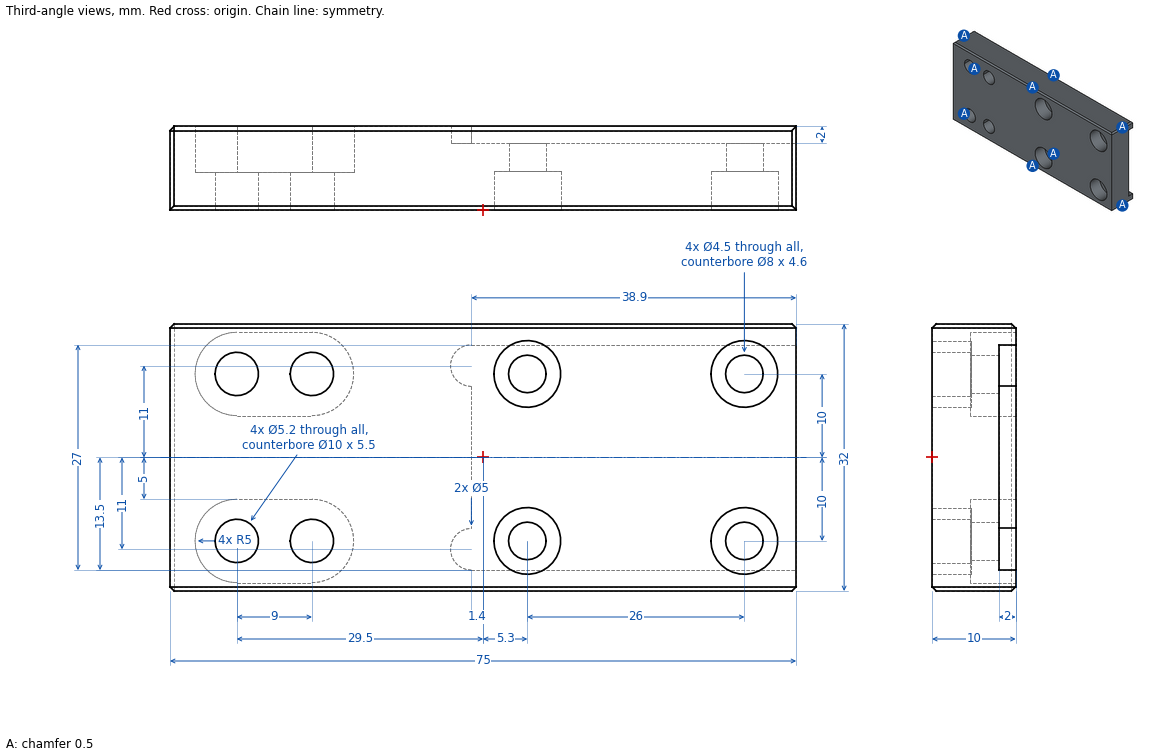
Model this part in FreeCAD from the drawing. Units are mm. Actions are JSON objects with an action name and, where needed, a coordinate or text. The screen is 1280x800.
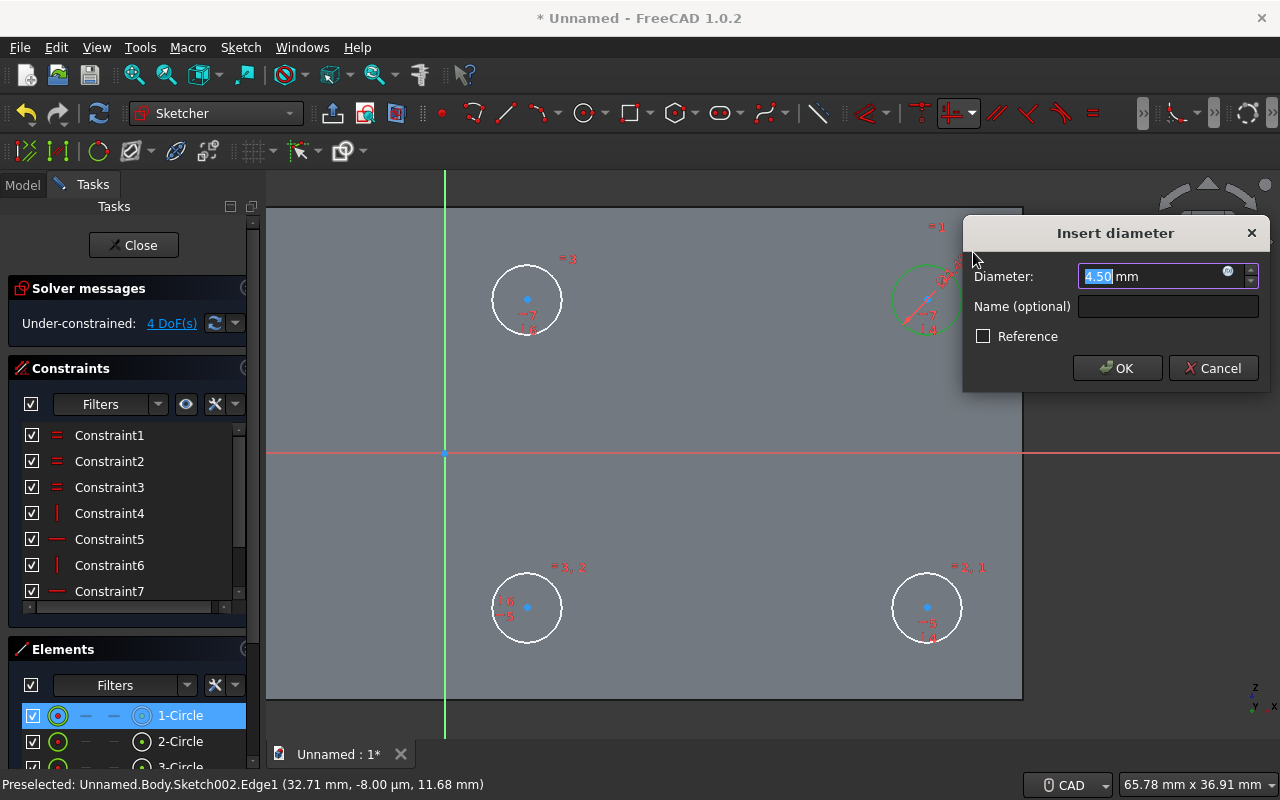
{"action": "type", "text": "4.5"}
{"action": "key", "text": "Return"}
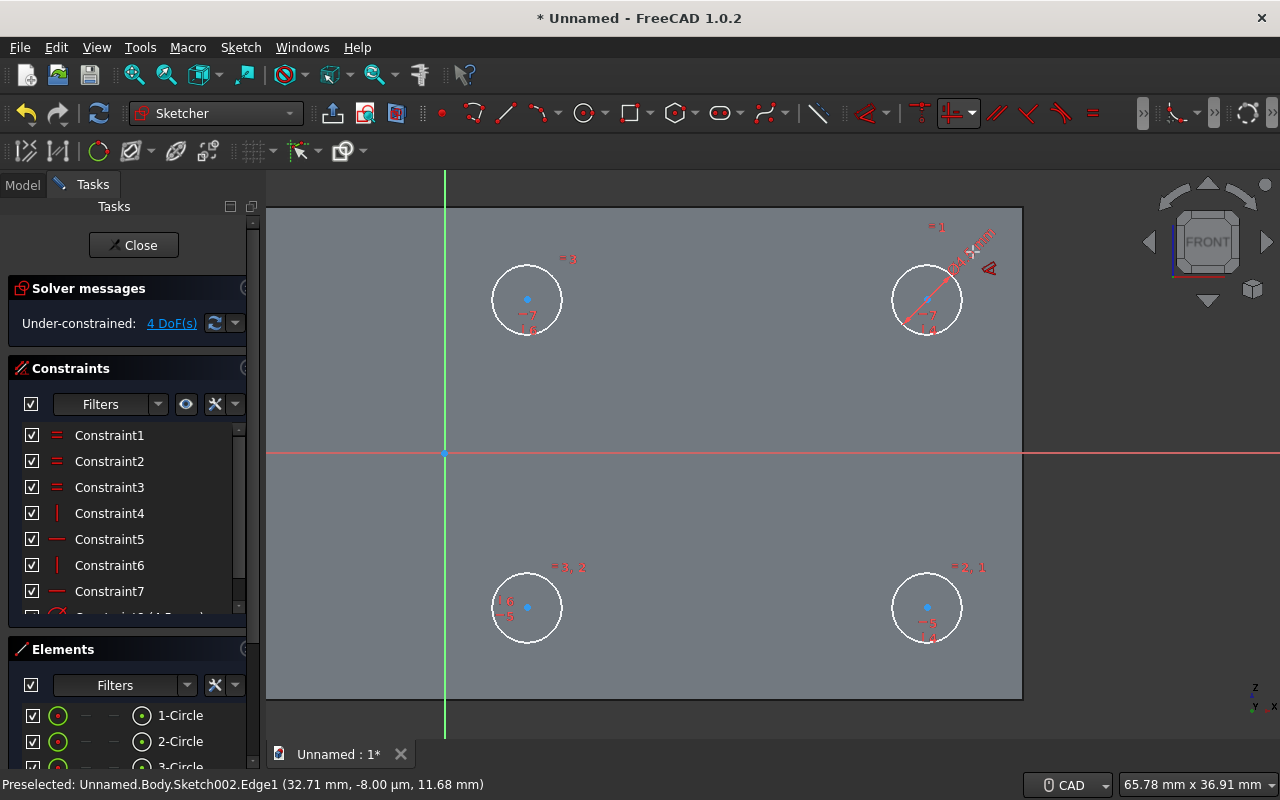
{"action": "left_click", "coordinate": [927, 300]}
{"action": "left_click", "coordinate": [411, 377]}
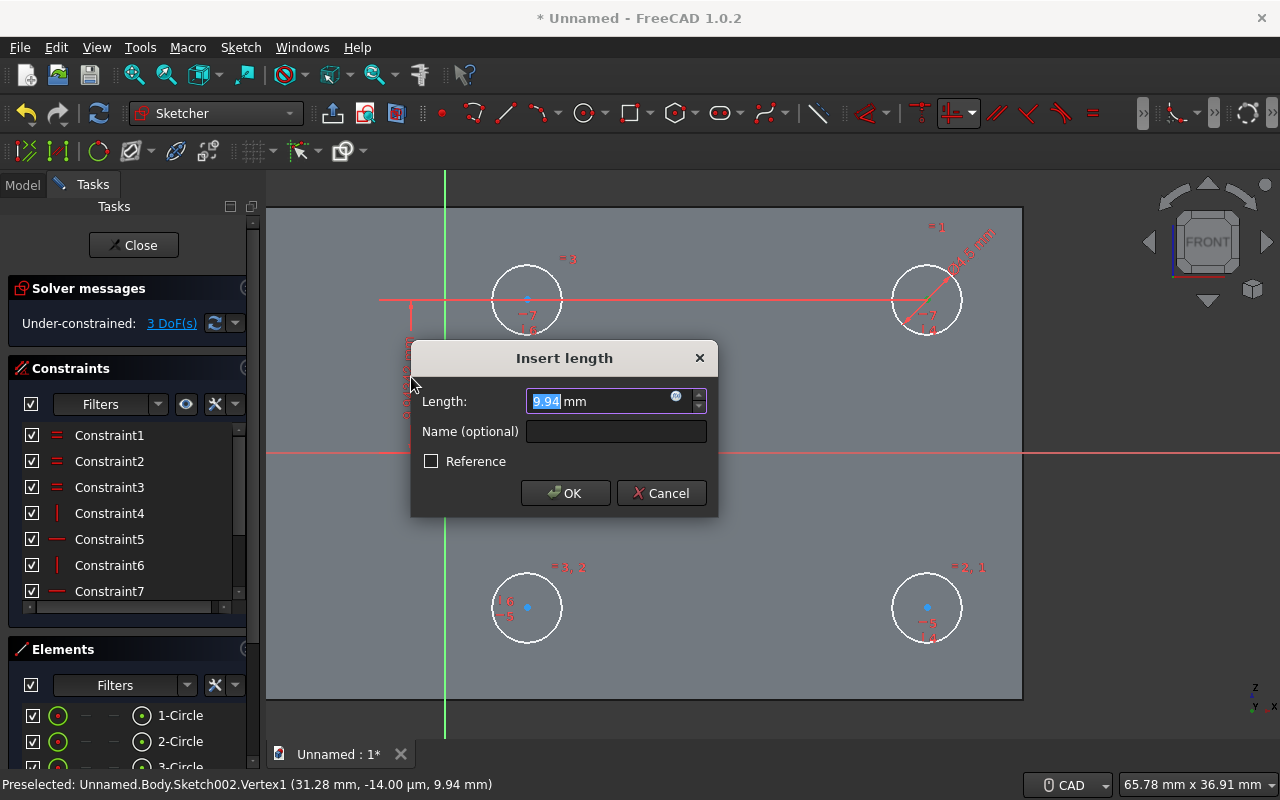
{"action": "type", "text": "10"}
{"action": "key", "text": "Return"}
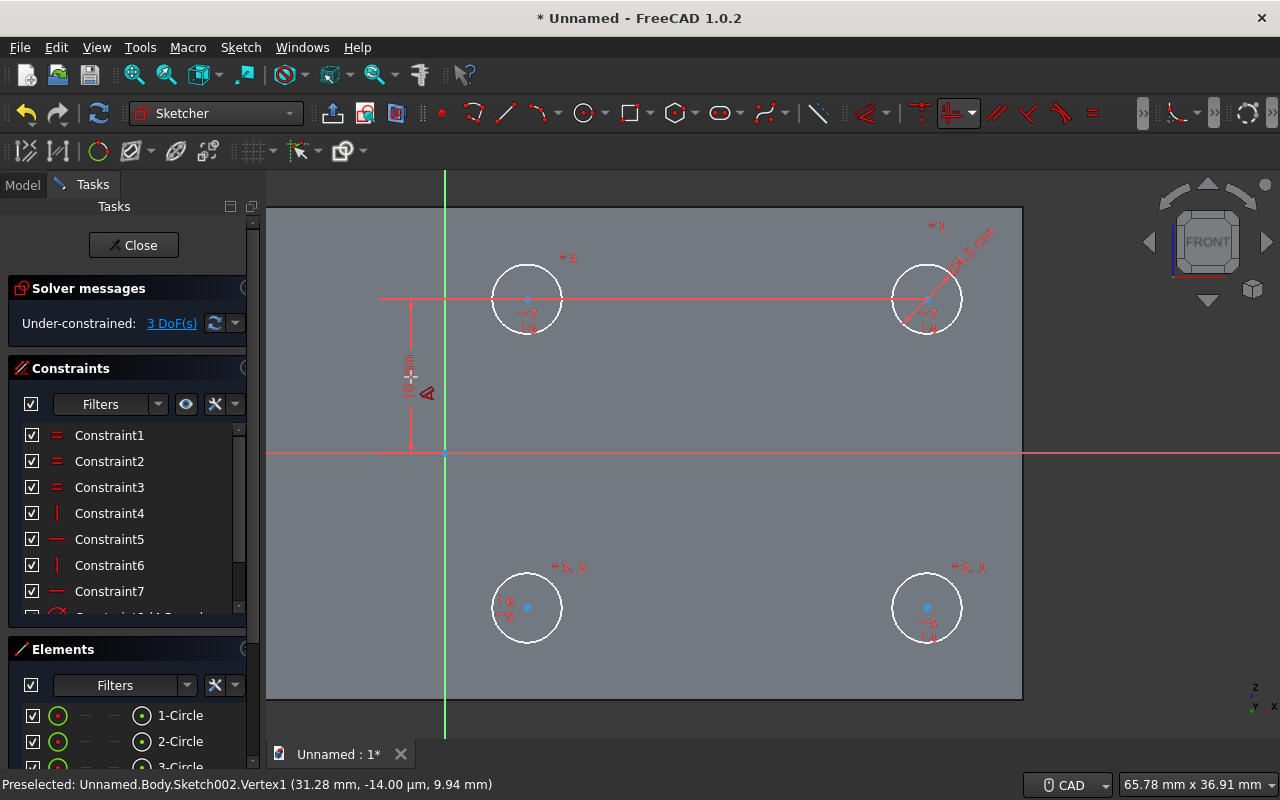
{"action": "left_click", "coordinate": [927, 608]}
{"action": "left_click", "coordinate": [411, 531]}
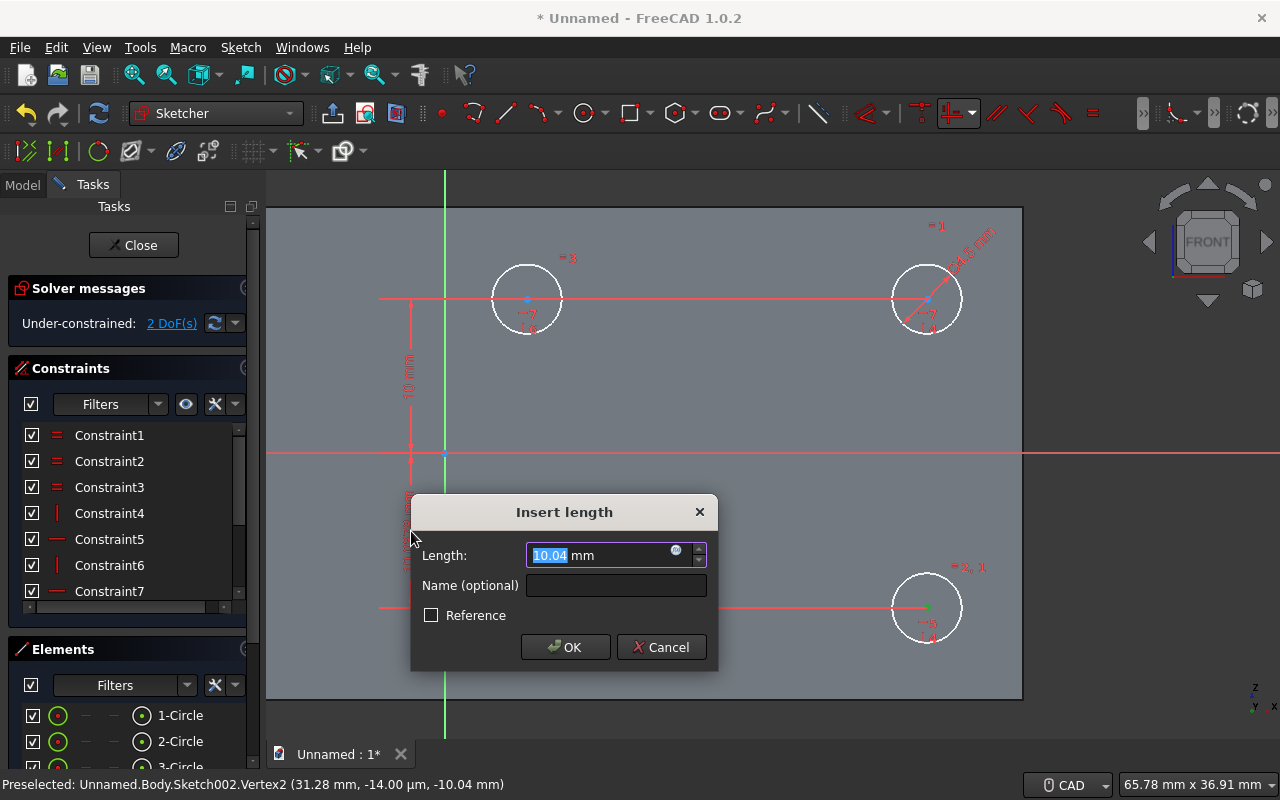
{"action": "type", "text": "10"}
{"action": "key", "text": "Return"}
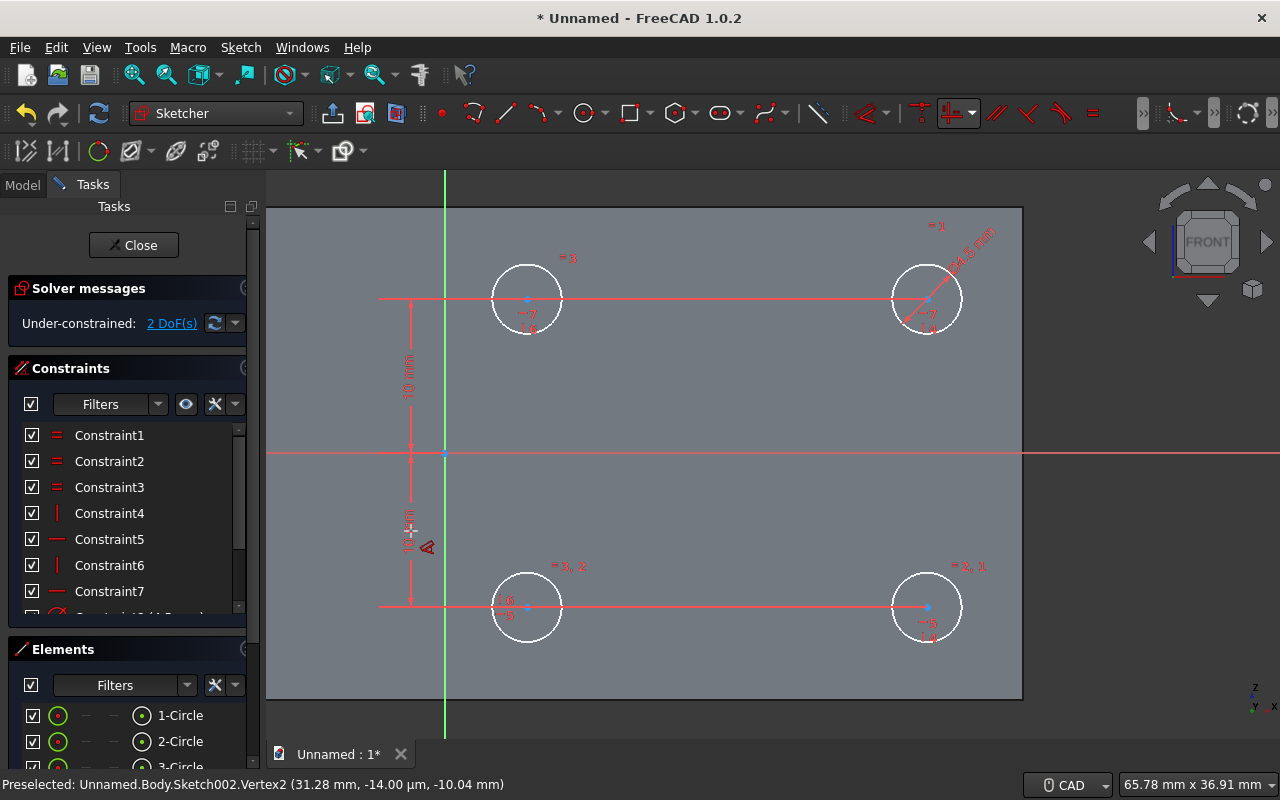
{"action": "left_click", "coordinate": [527, 607]}
{"action": "left_click", "coordinate": [486, 641]}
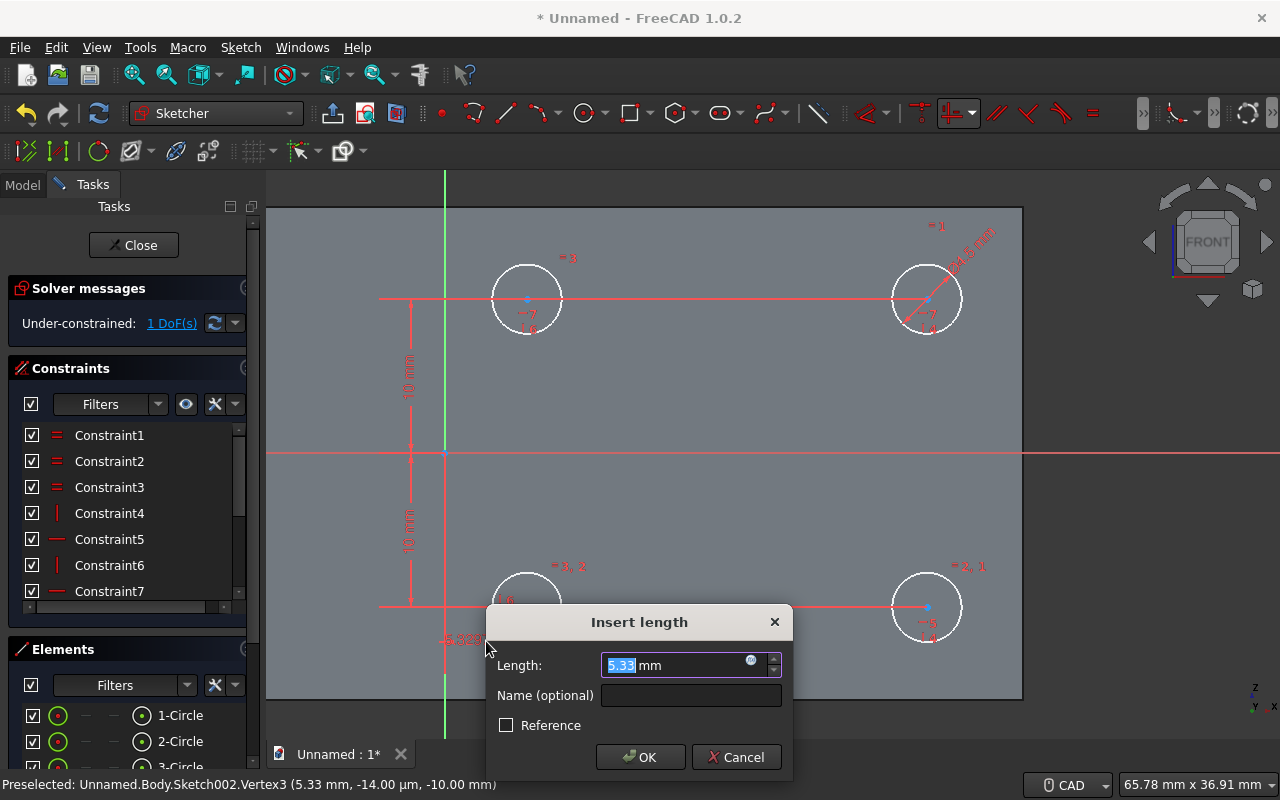
{"action": "type", "text": "5.3"}
{"action": "key", "text": "Return"}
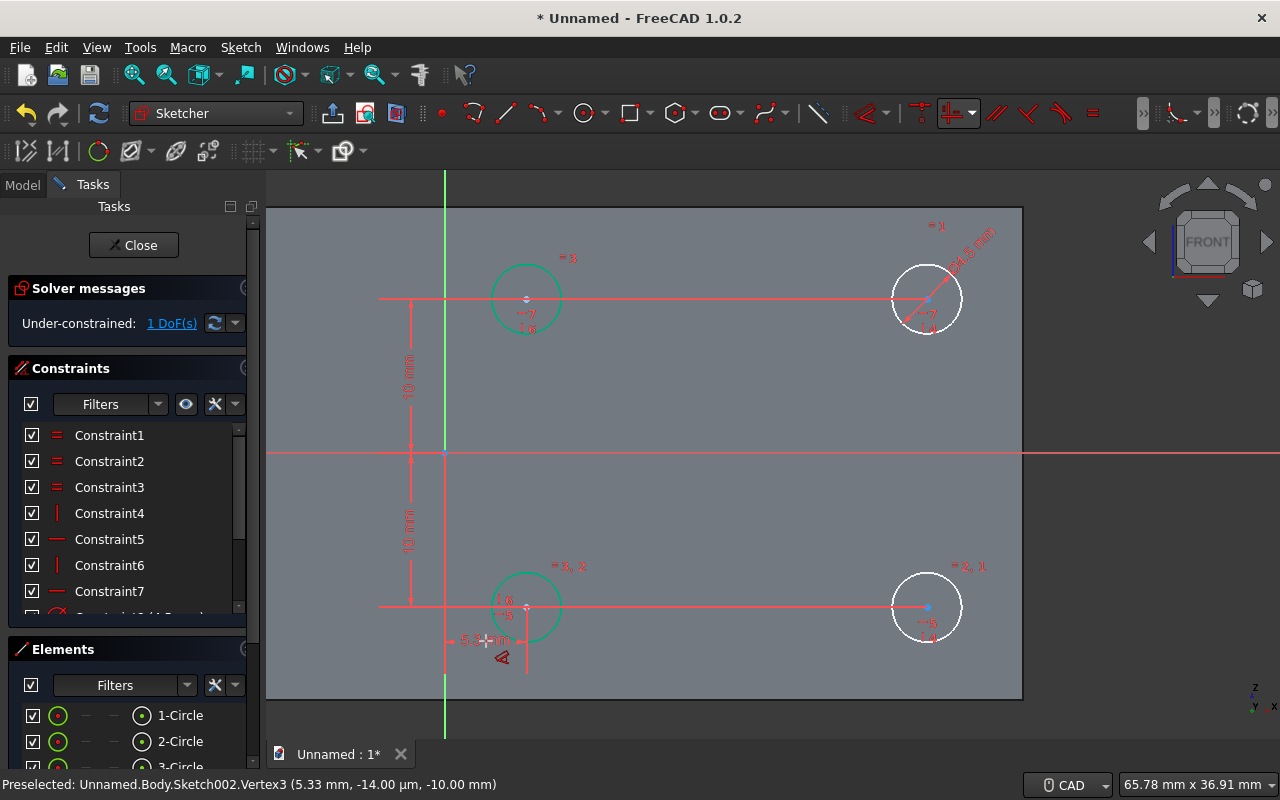
{"action": "left_click", "coordinate": [927, 607]}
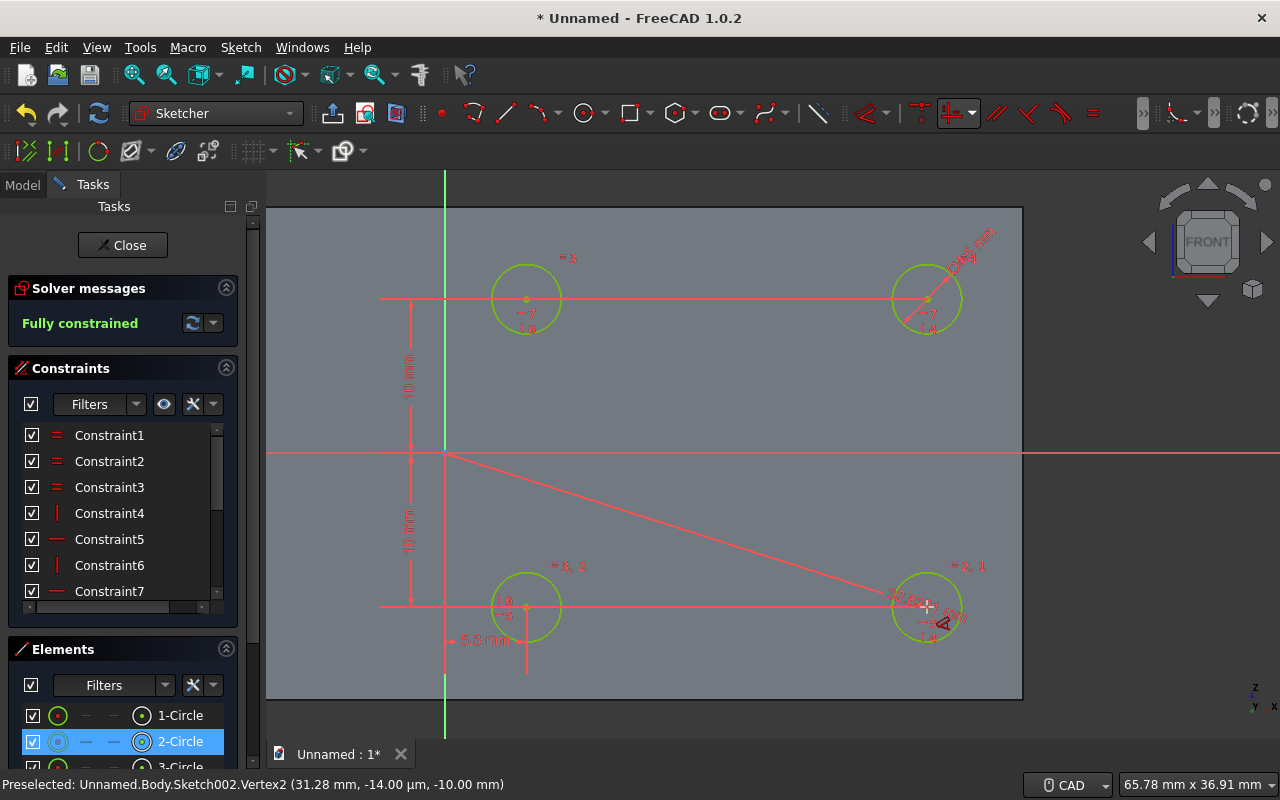
{"action": "left_click", "coordinate": [527, 607]}
{"action": "left_click", "coordinate": [727, 641]}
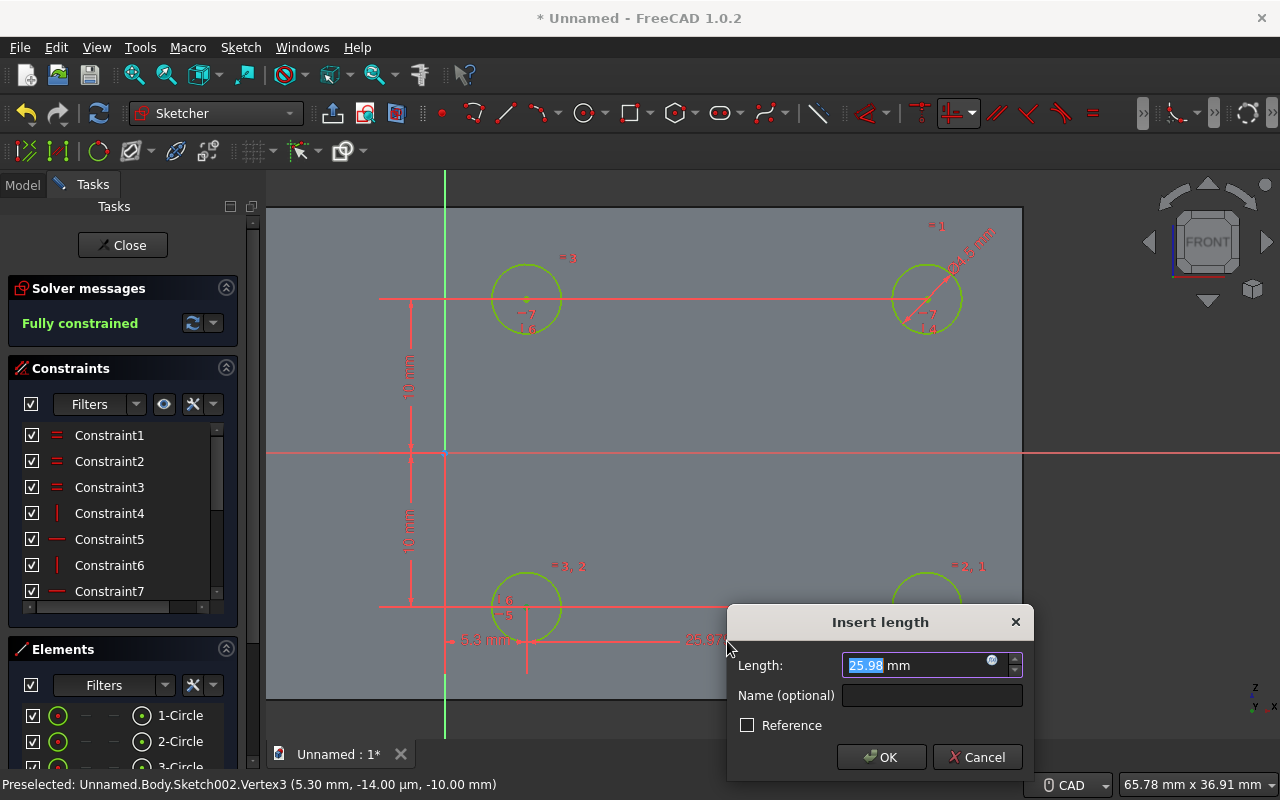
{"action": "type", "text": "26"}
{"action": "key", "text": "Return"}
{"action": "key", "text": "Escape"}